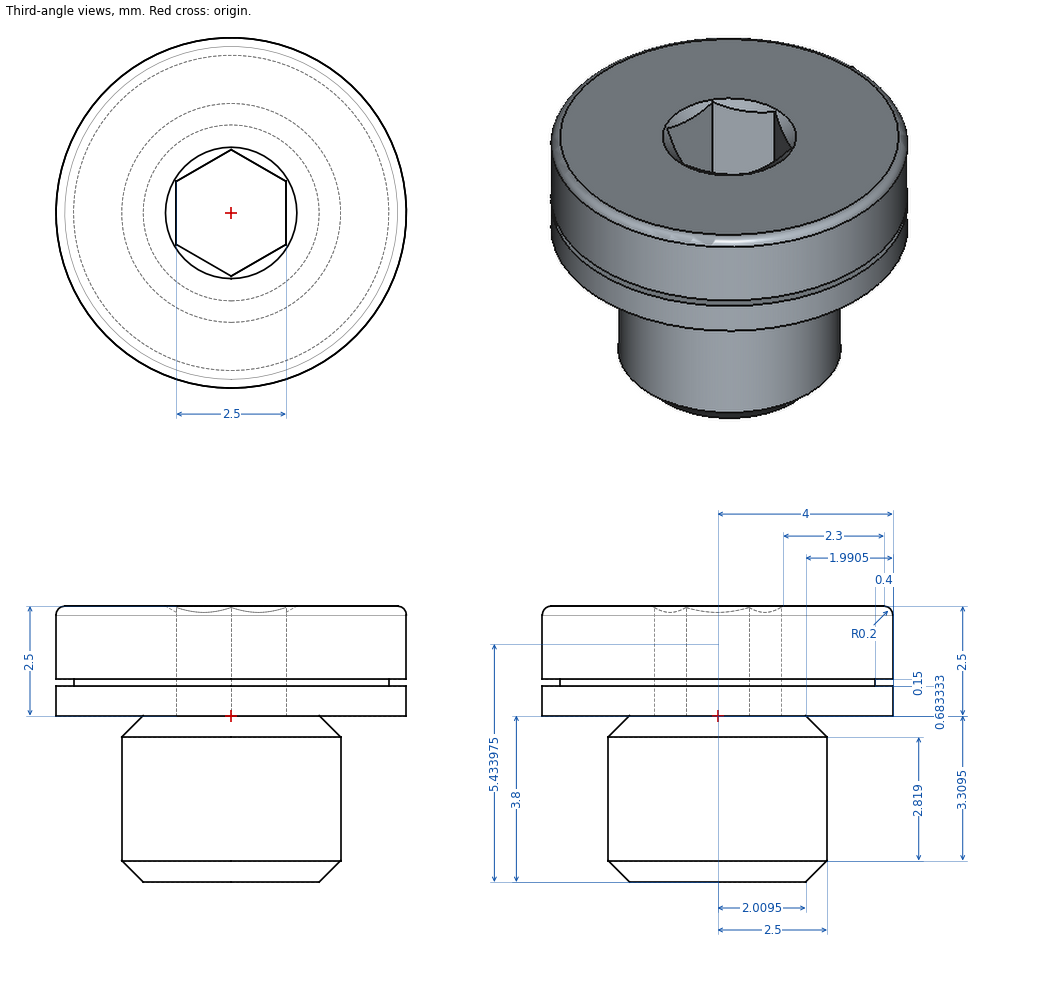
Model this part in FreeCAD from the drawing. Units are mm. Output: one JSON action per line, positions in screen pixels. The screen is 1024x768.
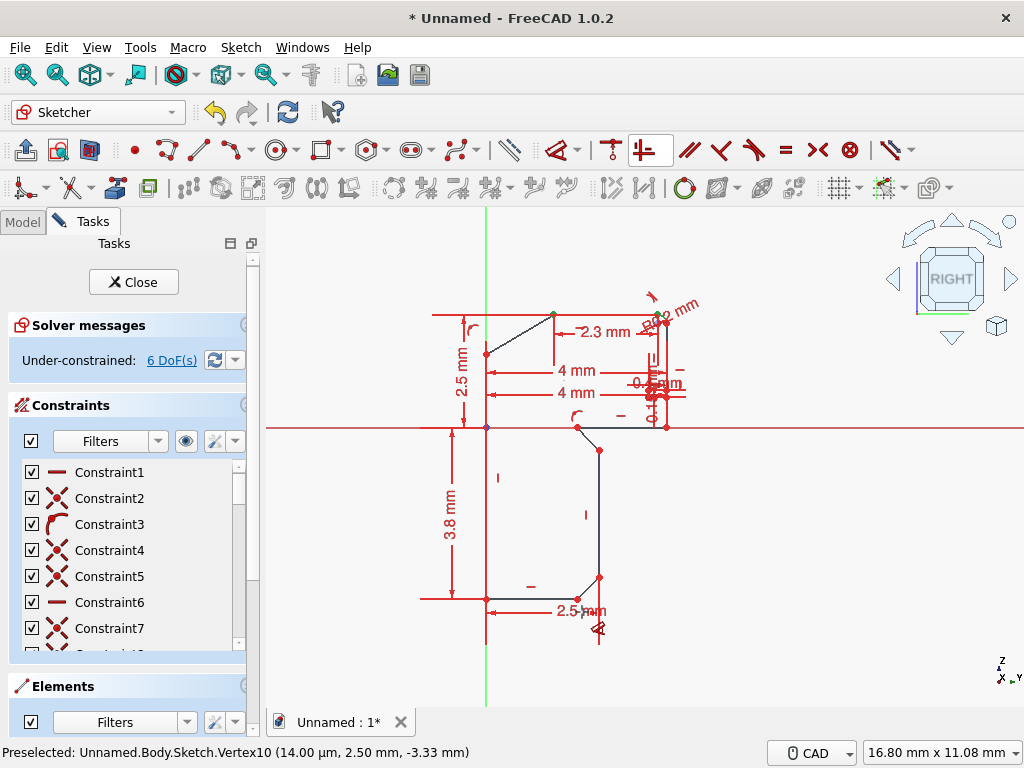
{"action": "left_click", "coordinate": [599, 540]}
{"action": "left_click", "coordinate": [633, 514]}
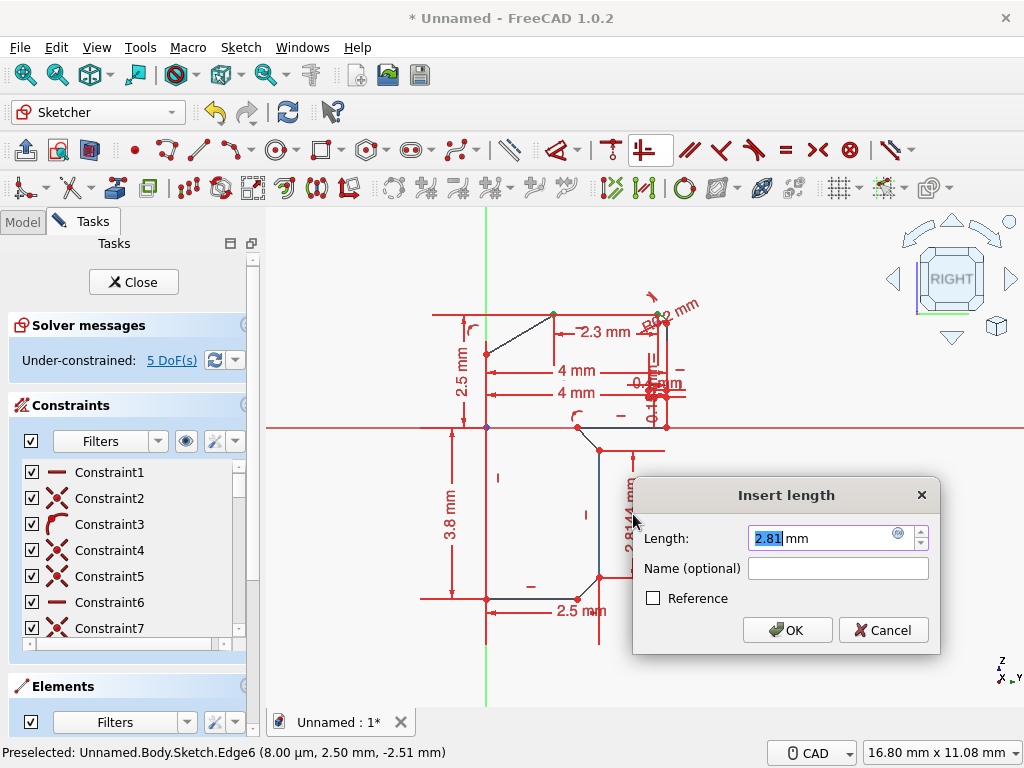
{"action": "type", "text": "2.819"}
{"action": "key", "text": "Return"}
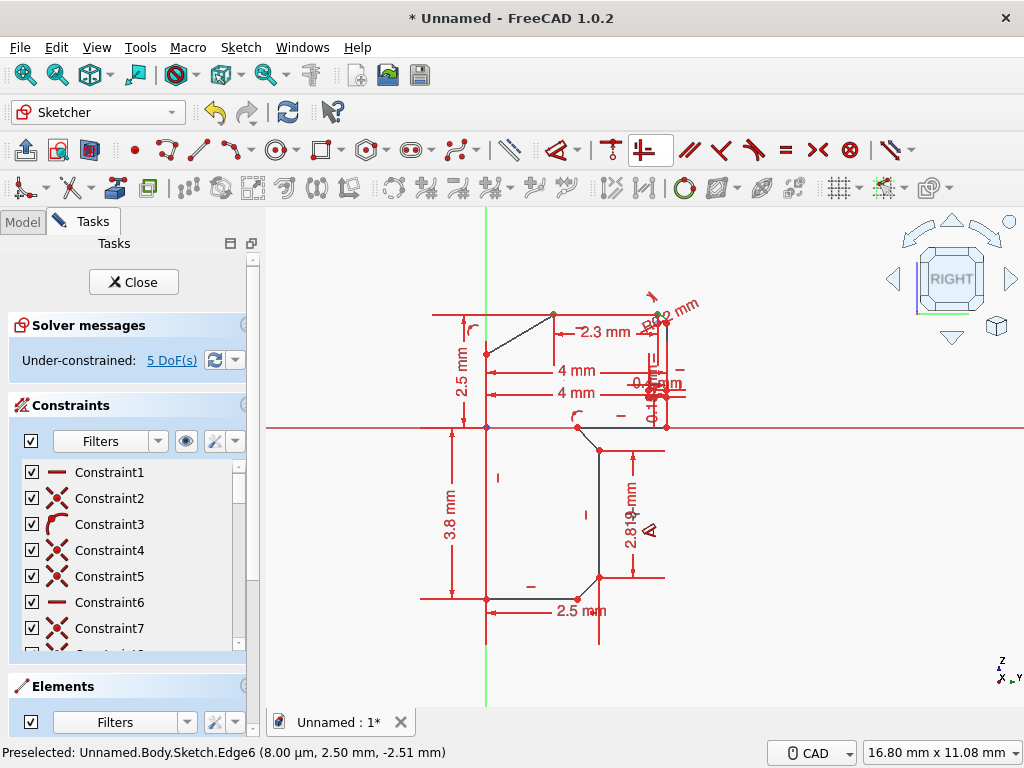
{"action": "left_click", "coordinate": [513, 599]}
{"action": "left_click", "coordinate": [532, 633]}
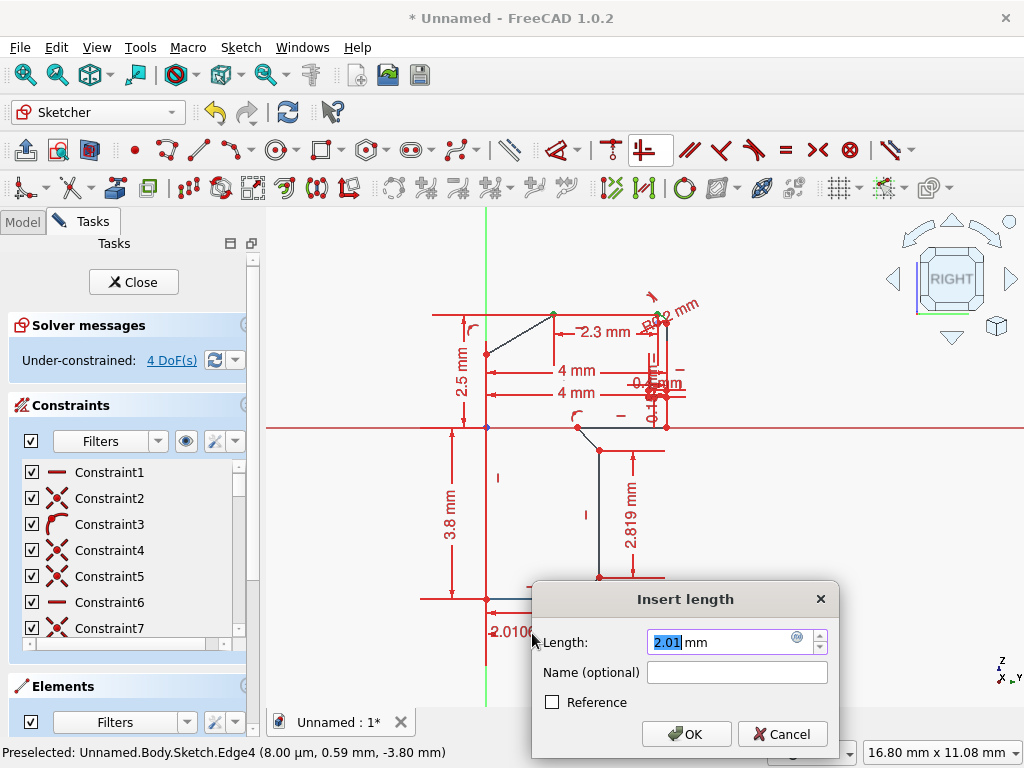
{"action": "type", "text": "2.0095"}
{"action": "key", "text": "Return"}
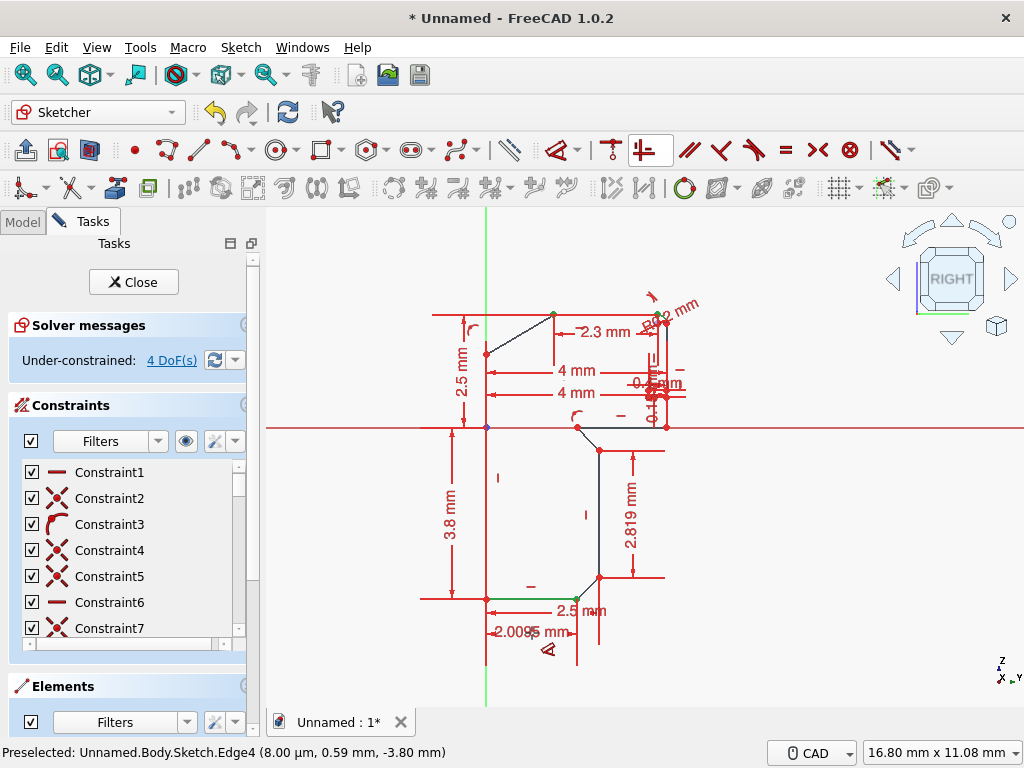
{"action": "left_click", "coordinate": [604, 428]}
{"action": "left_click", "coordinate": [622, 462]}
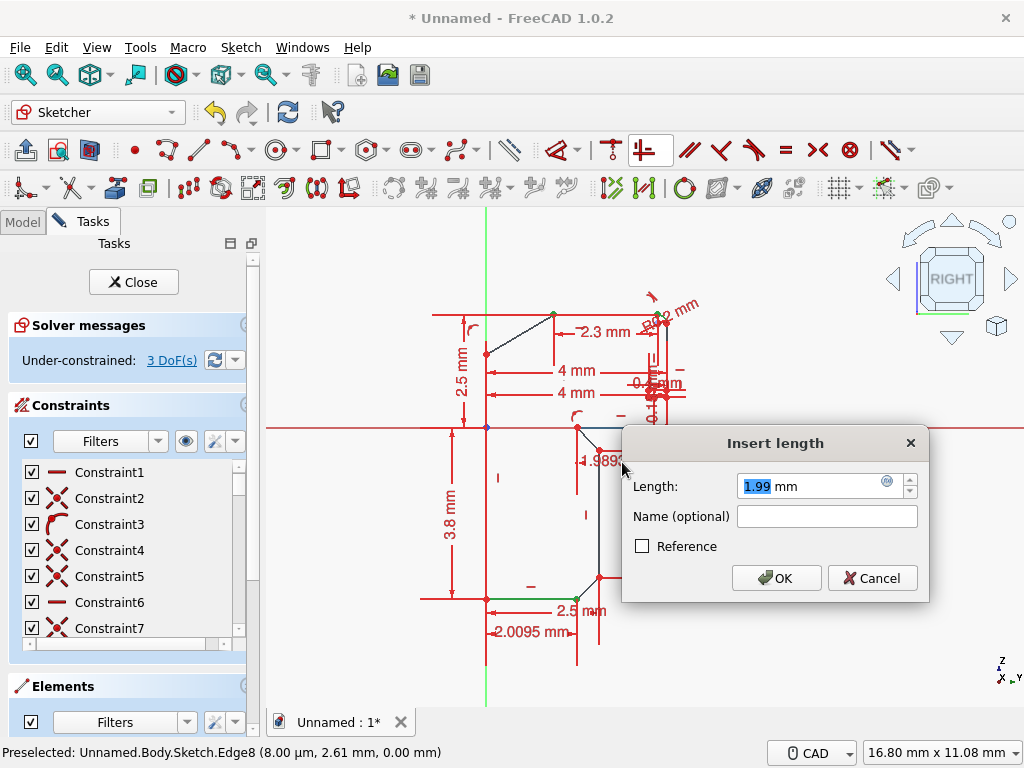
{"action": "type", "text": "1.9905"}
{"action": "key", "text": "Return"}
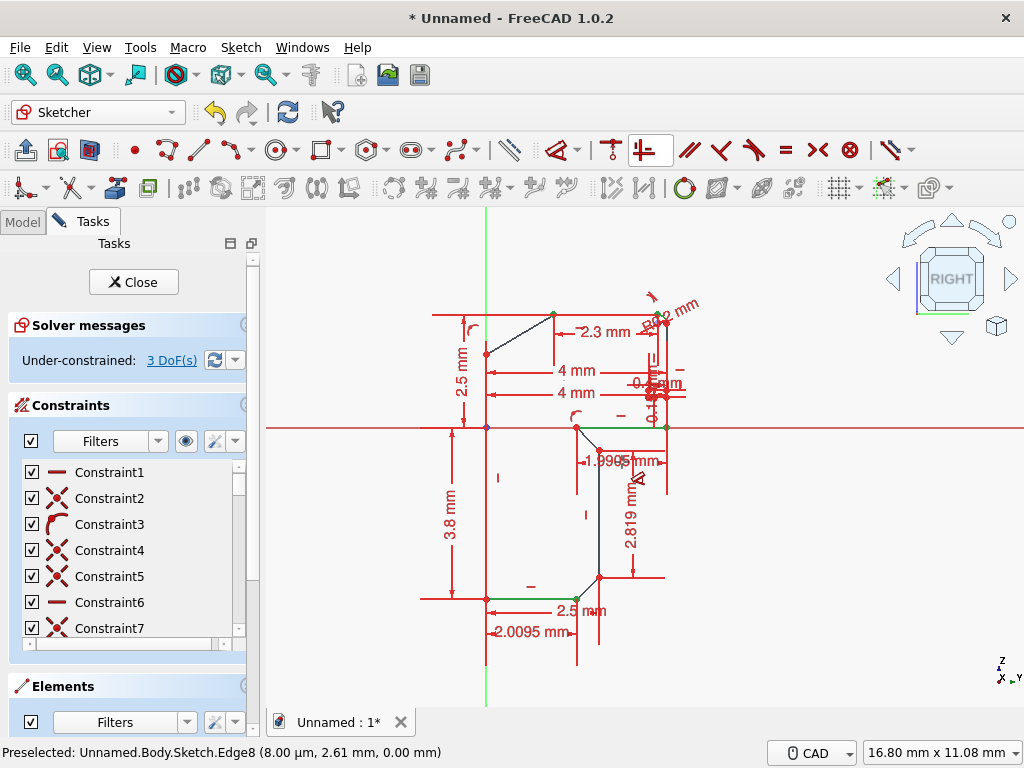
{"action": "left_click", "coordinate": [599, 578]}
{"action": "left_click", "coordinate": [452, 468]}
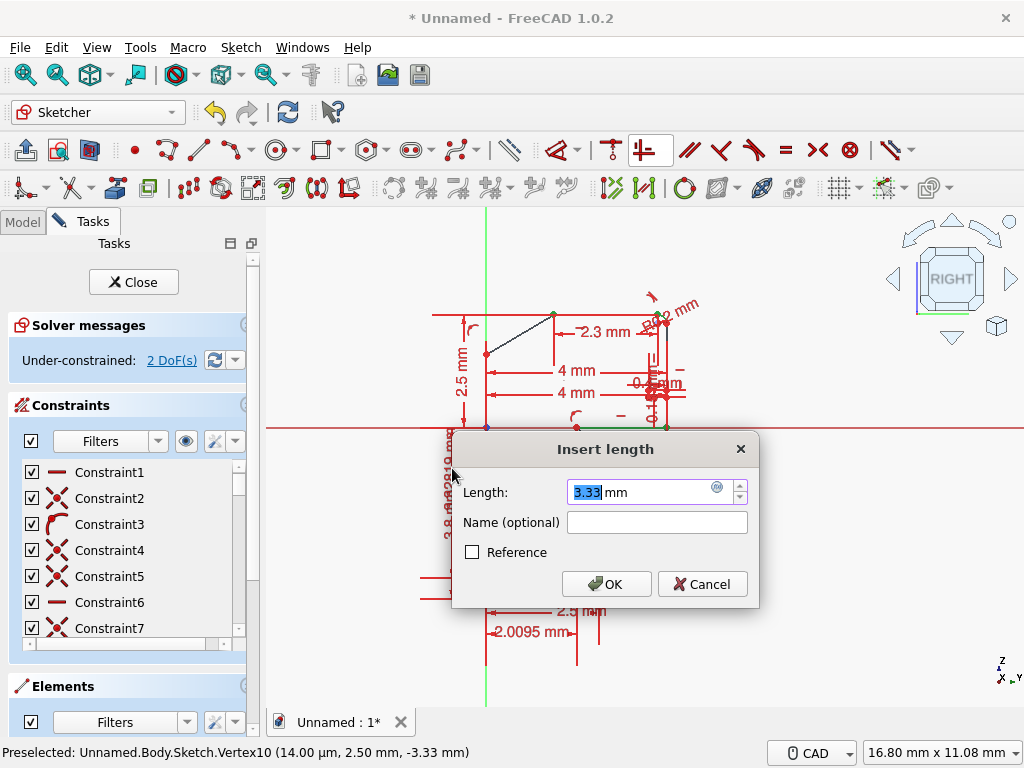
{"action": "type", "text": "3.3095"}
{"action": "key", "text": "Return"}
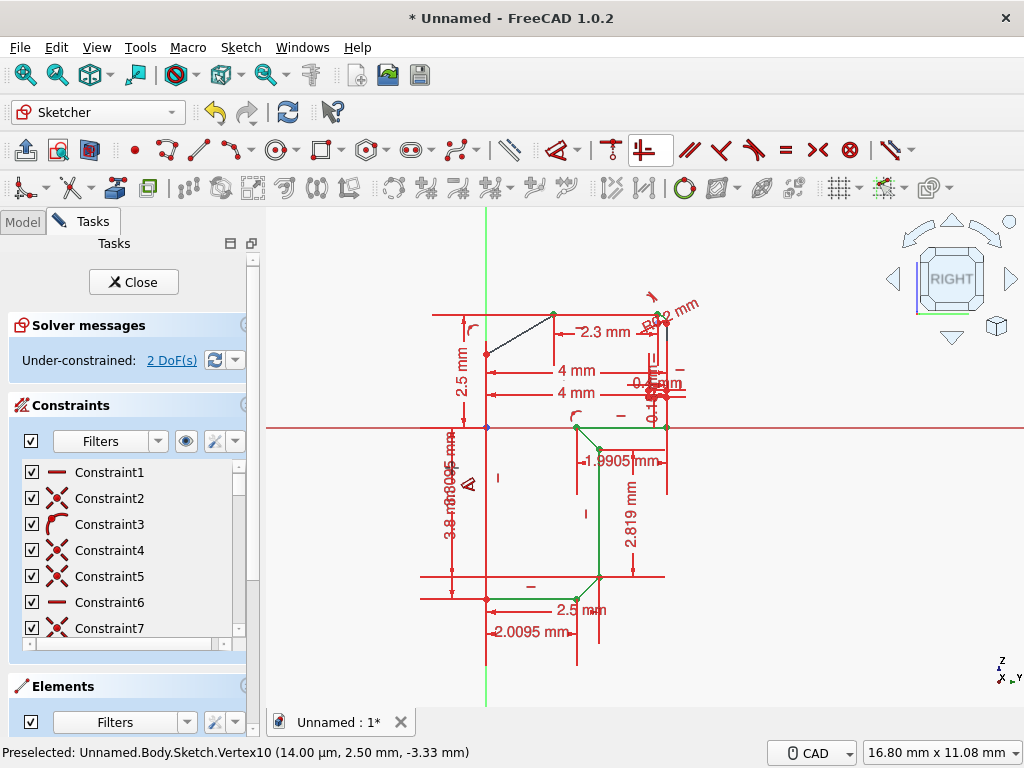
{"action": "left_click", "coordinate": [486, 526]}
{"action": "left_click", "coordinate": [452, 563]}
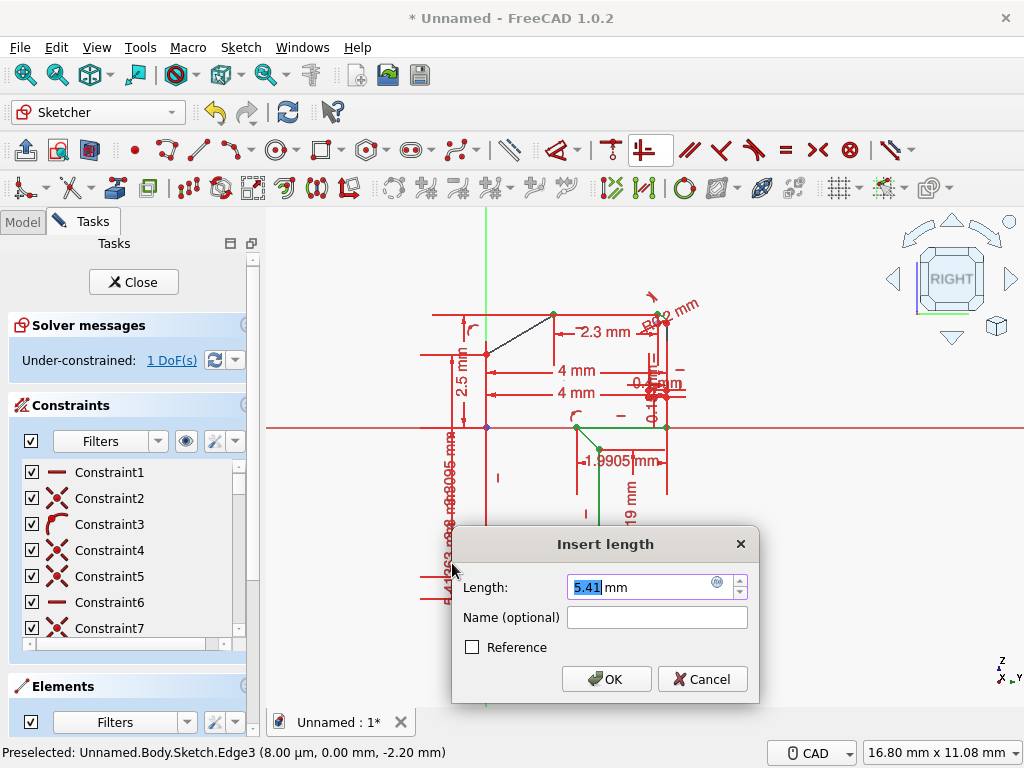
{"action": "type", "text": "5.433975"}
{"action": "key", "text": "Return"}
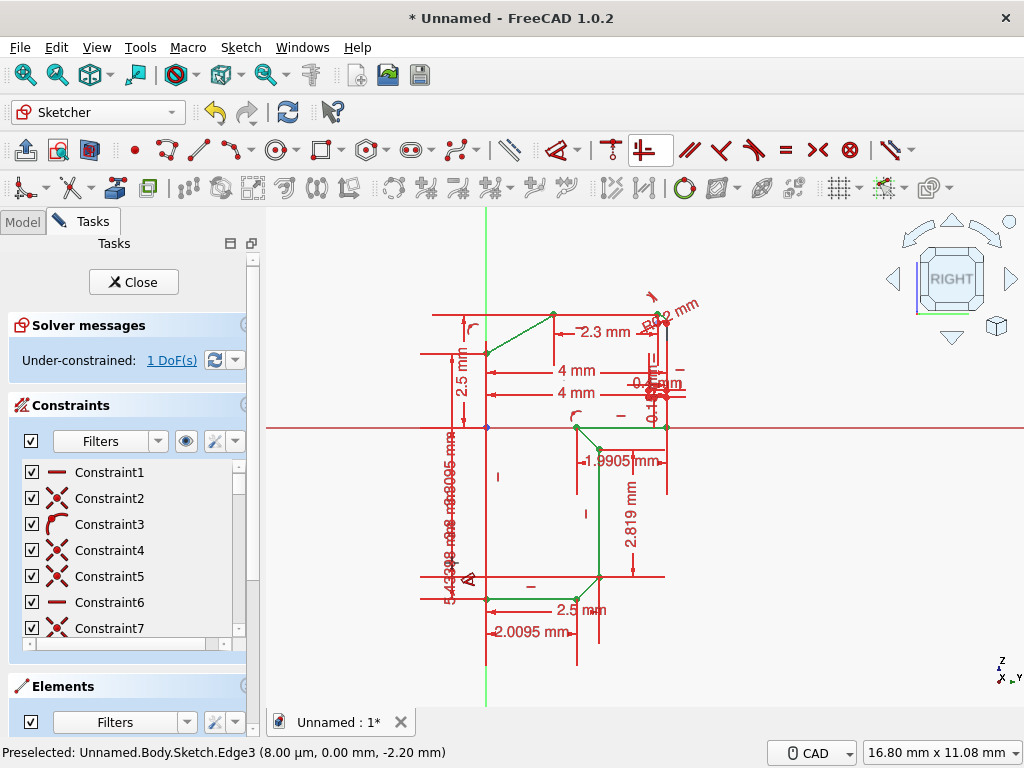
{"action": "scroll", "coordinate": [667, 419], "scroll_direction": "up", "scroll_amount": 3}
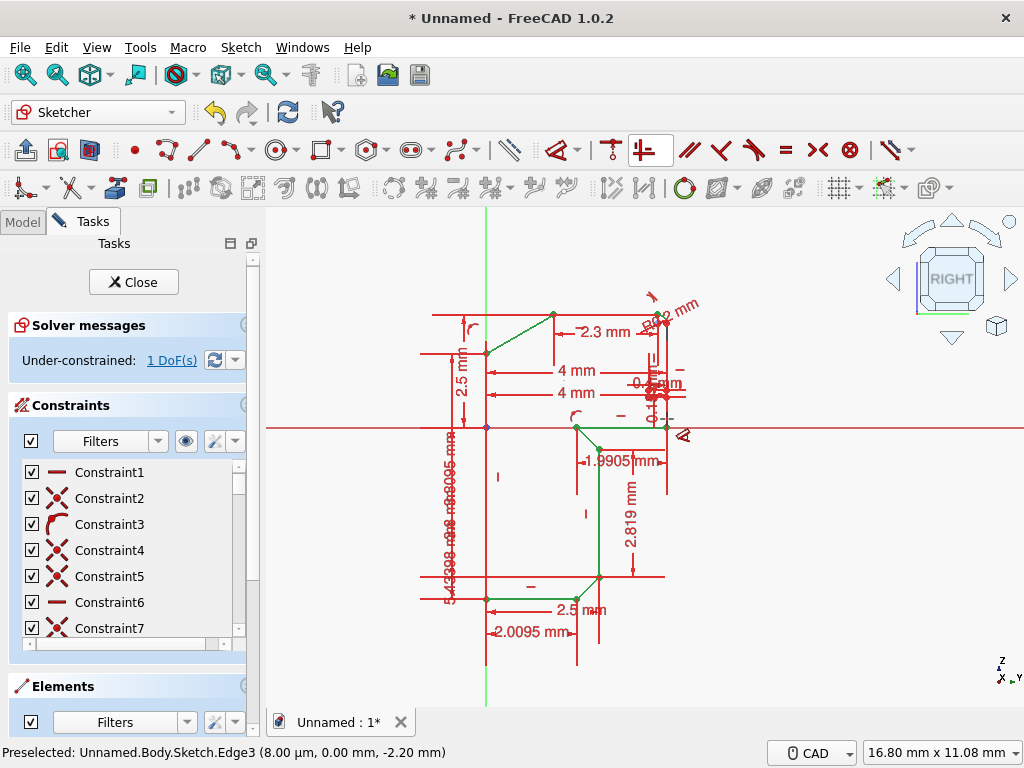
{"action": "left_click", "coordinate": [666, 418]}
{"action": "left_click", "coordinate": [700, 407]}